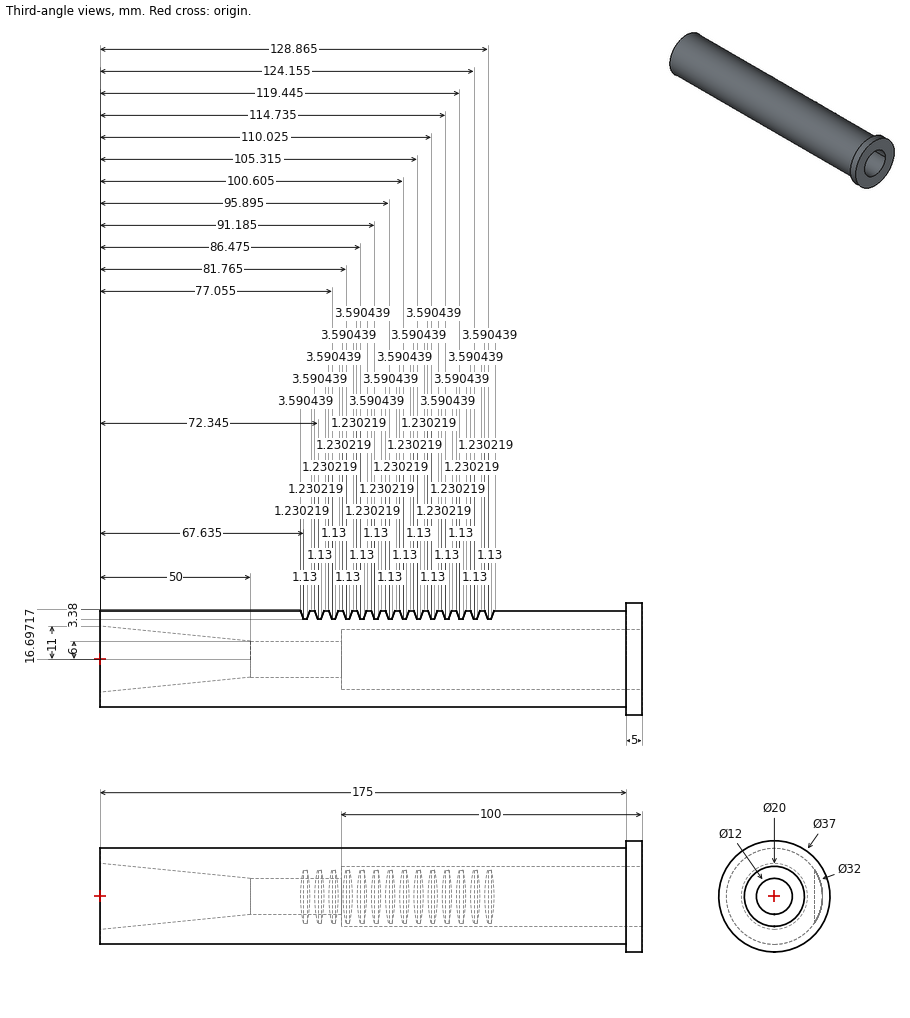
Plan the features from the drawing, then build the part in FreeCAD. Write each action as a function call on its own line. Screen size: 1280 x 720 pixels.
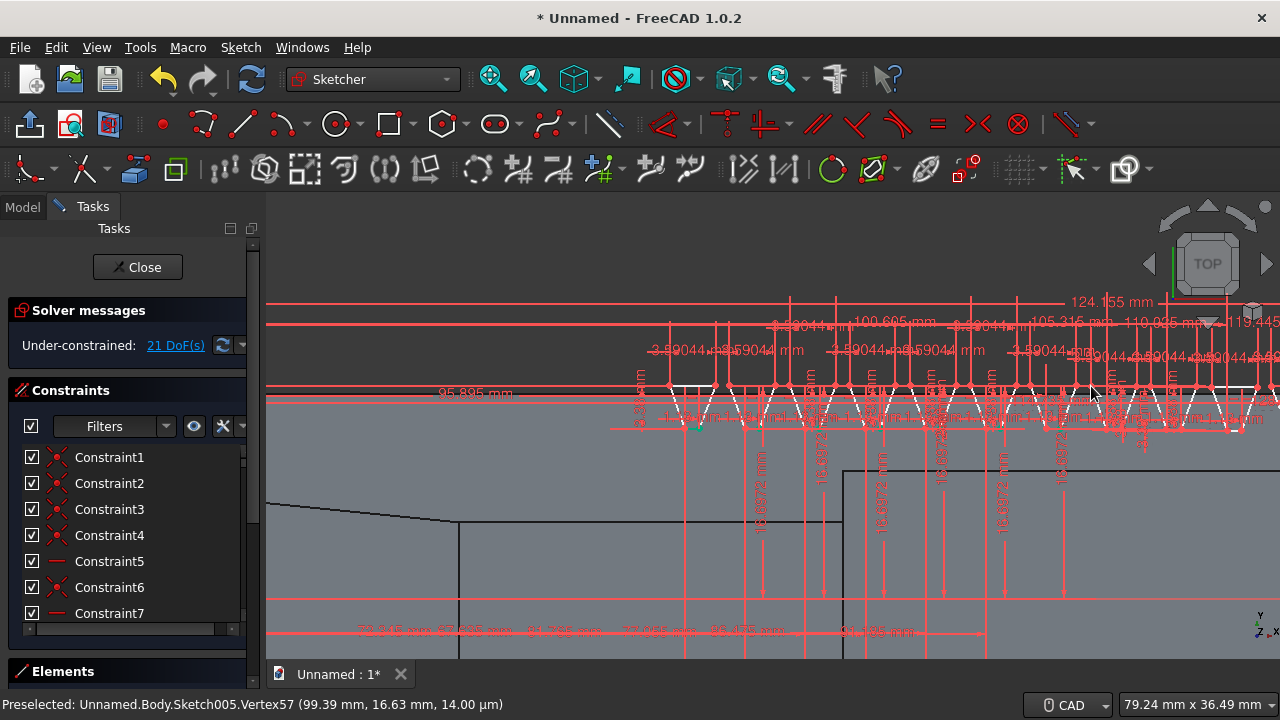
click(1091, 386)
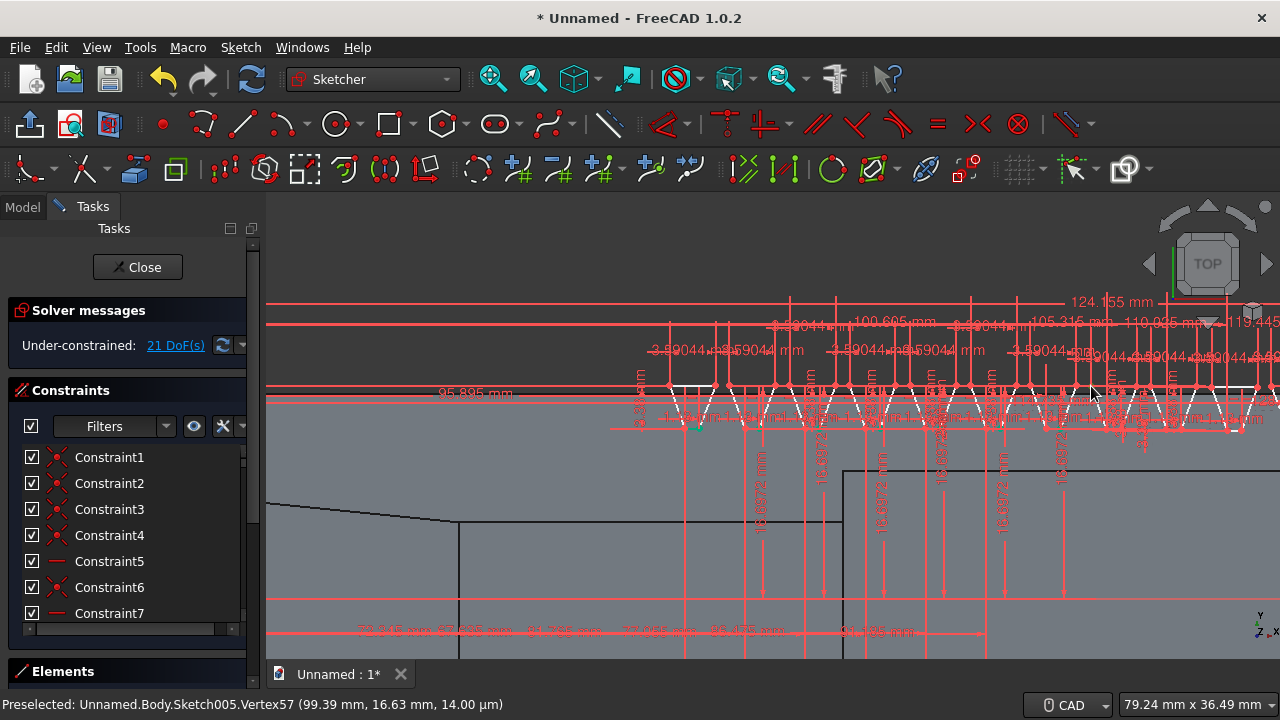
key(i)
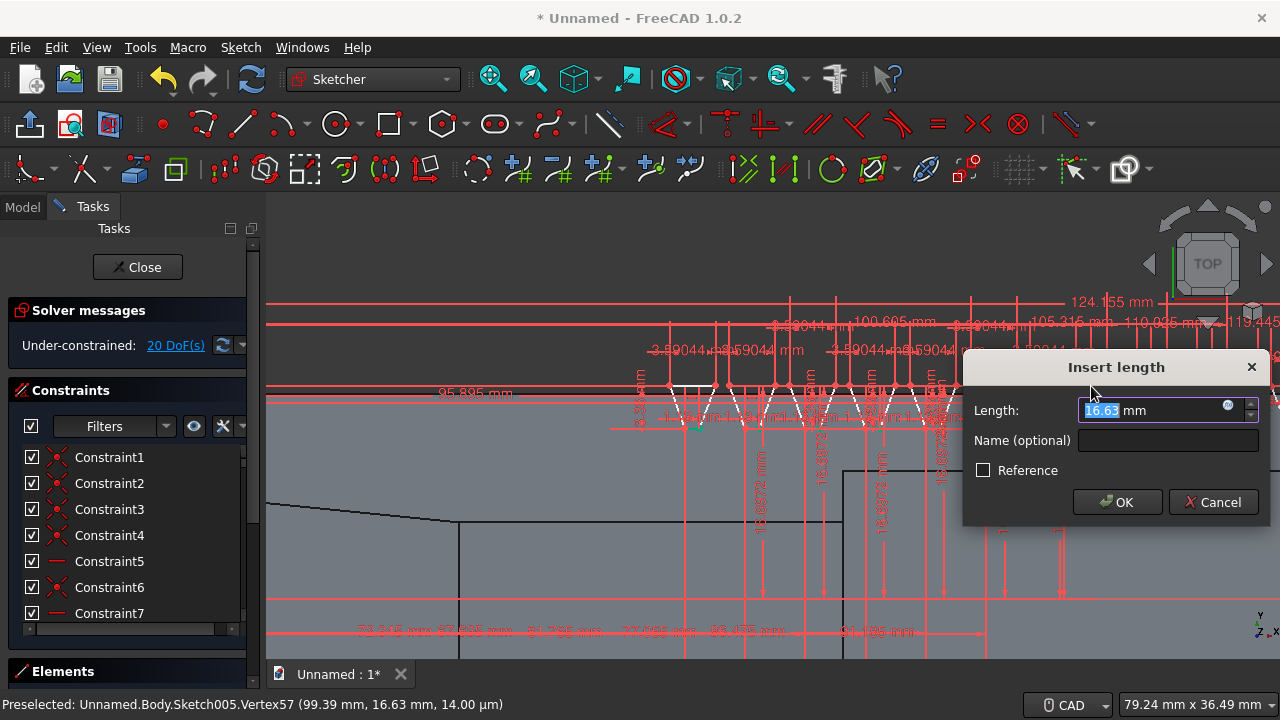
text(16.69717)
key(Return)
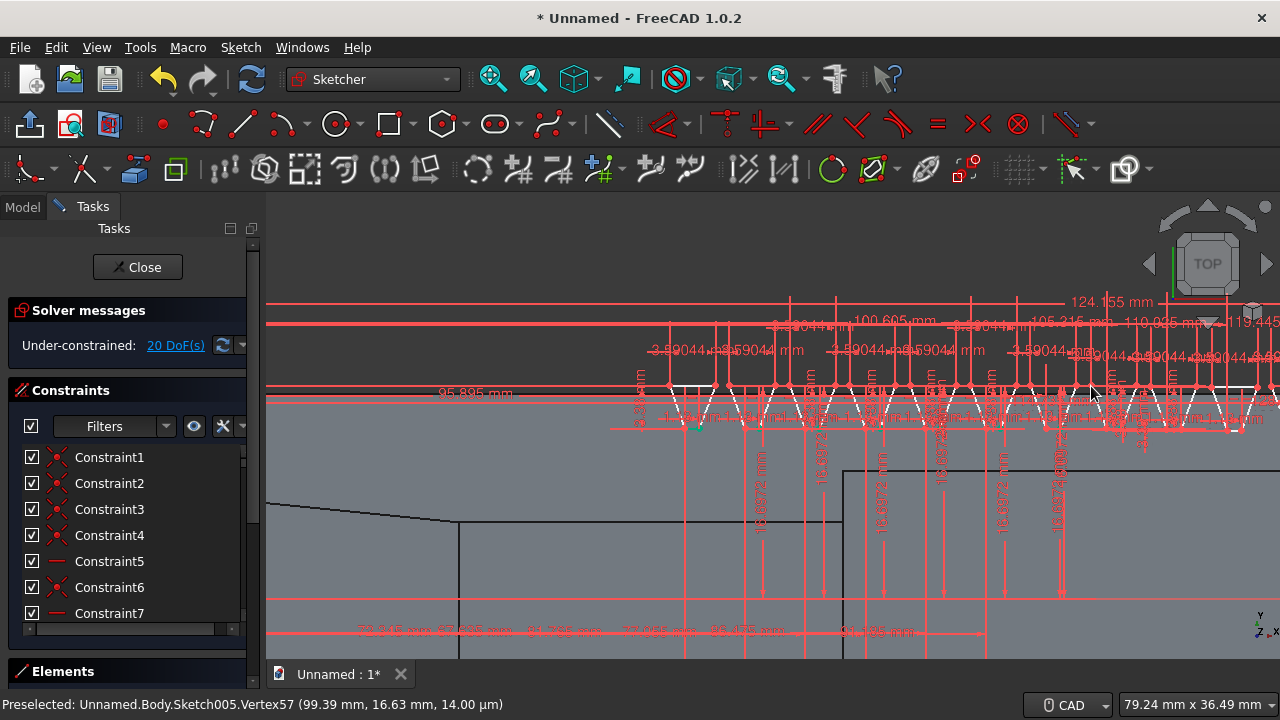
scroll(731, 387, down, 5)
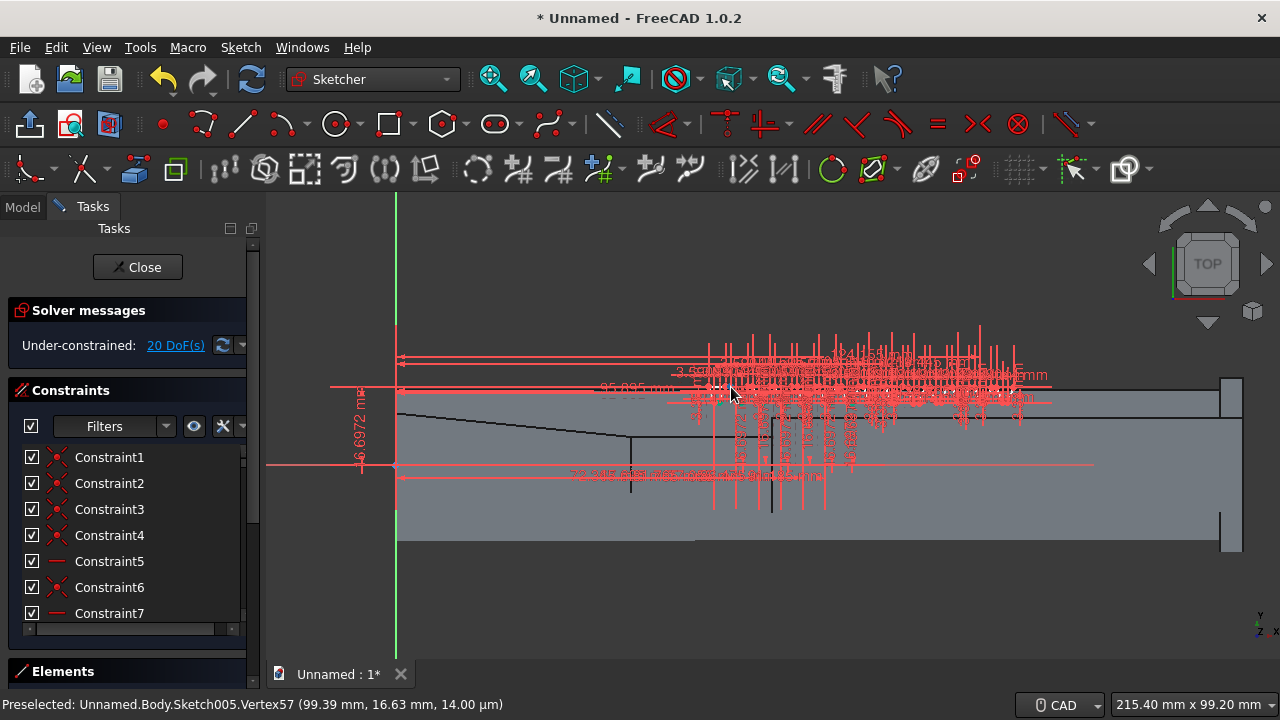
scroll(886, 387, up, 5)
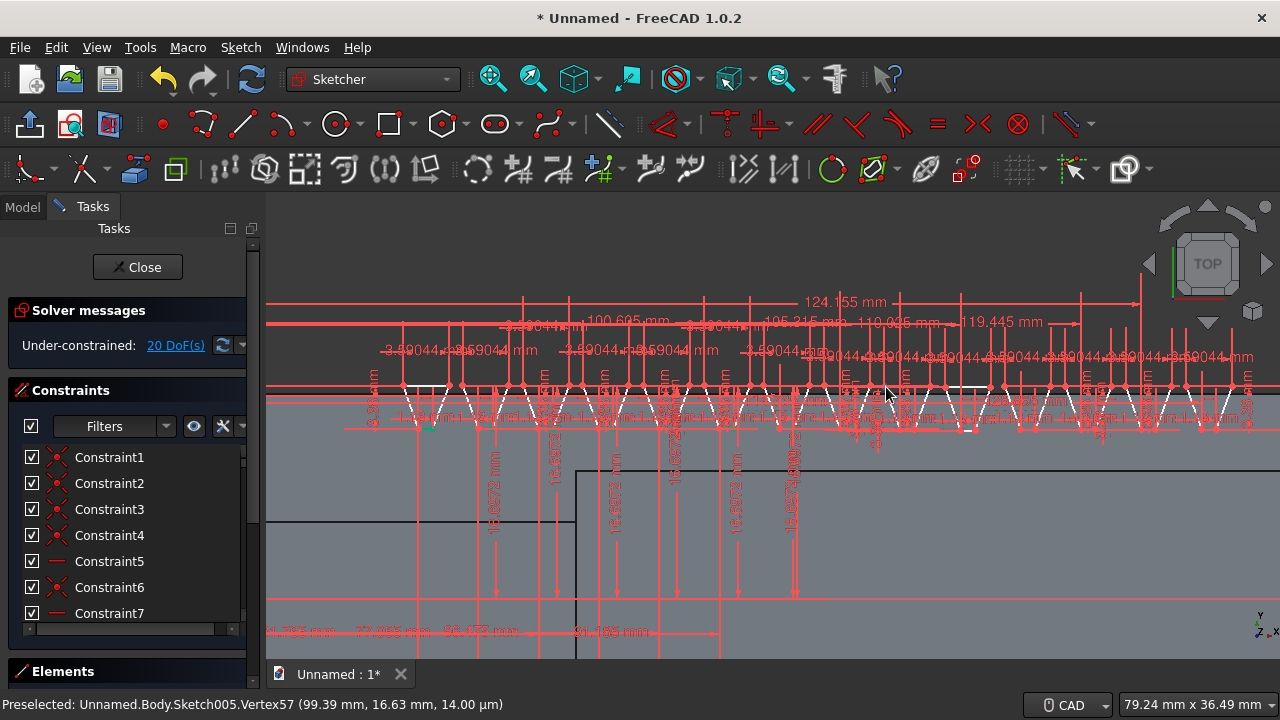
click(884, 386)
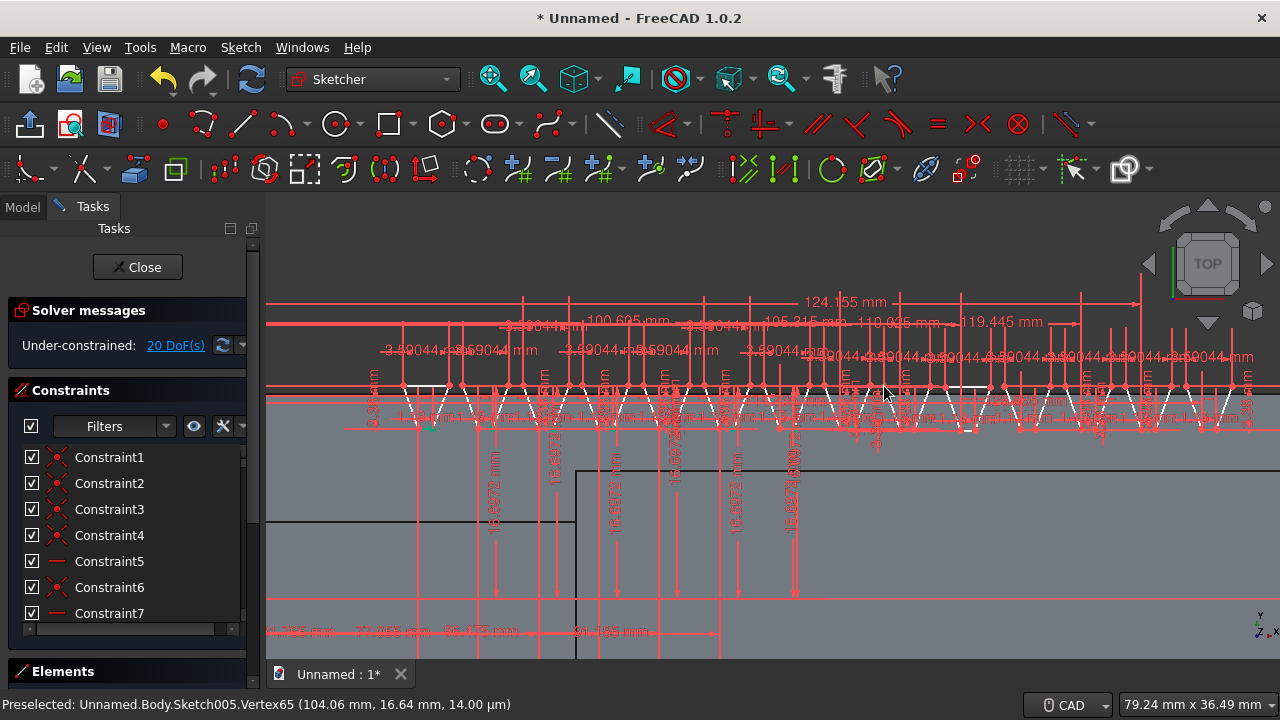
key(i)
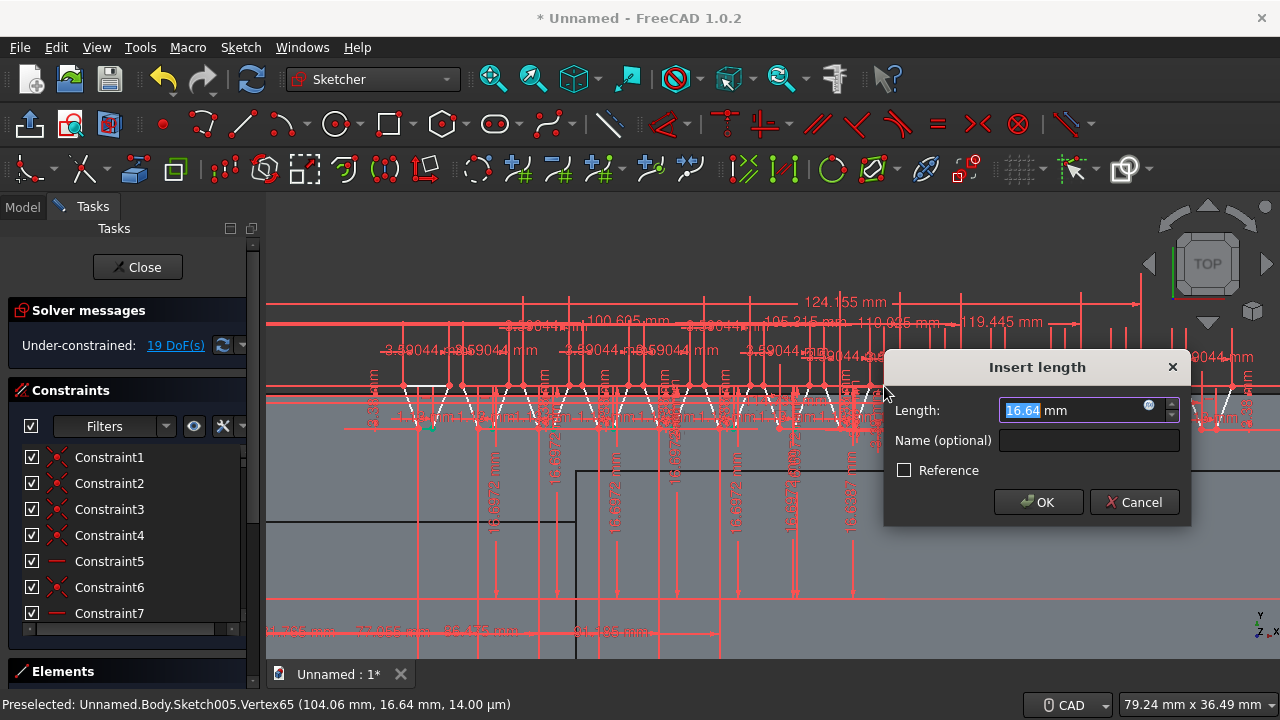
text(16.69717)
key(Return)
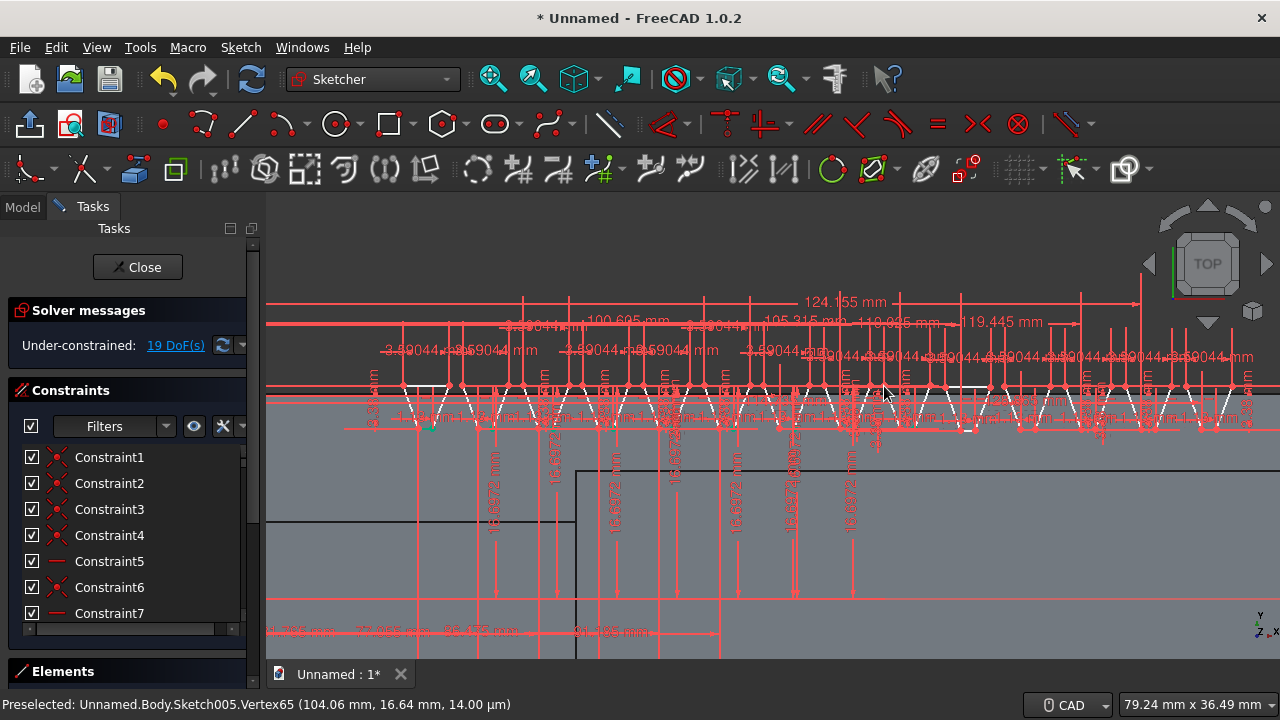
click(945, 387)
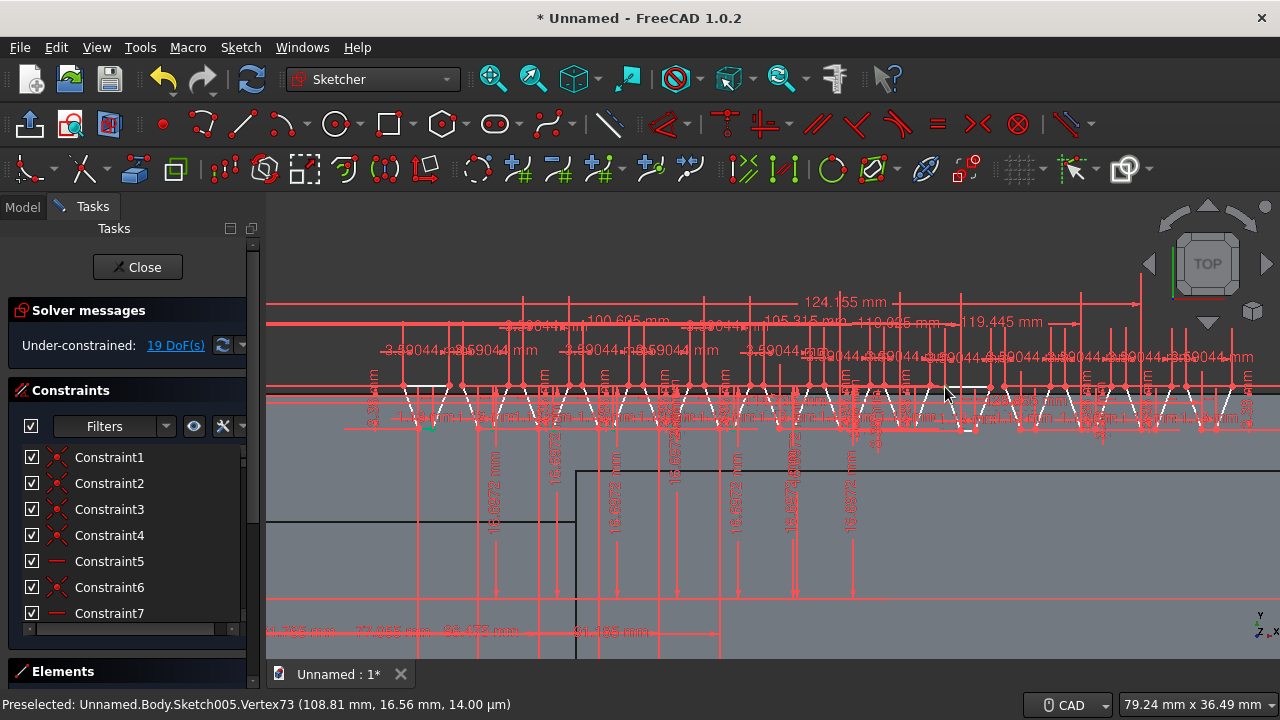
key(i)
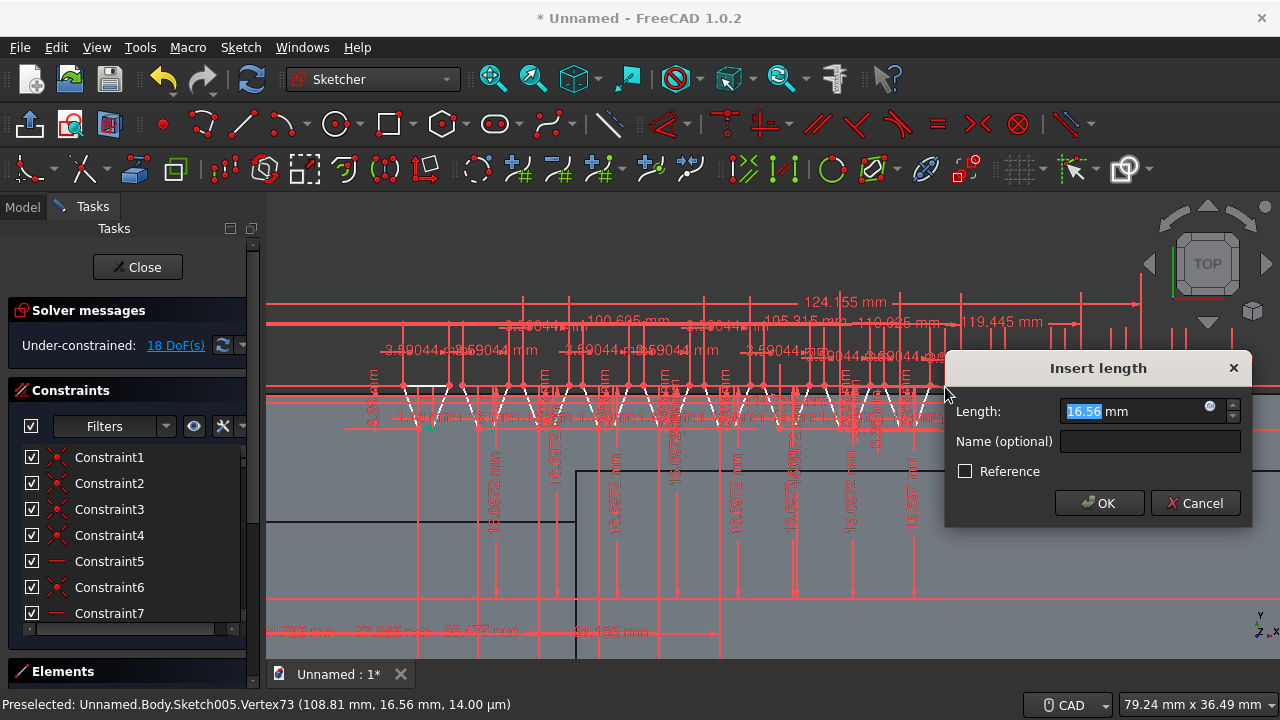
text(16.69717)
key(Return)